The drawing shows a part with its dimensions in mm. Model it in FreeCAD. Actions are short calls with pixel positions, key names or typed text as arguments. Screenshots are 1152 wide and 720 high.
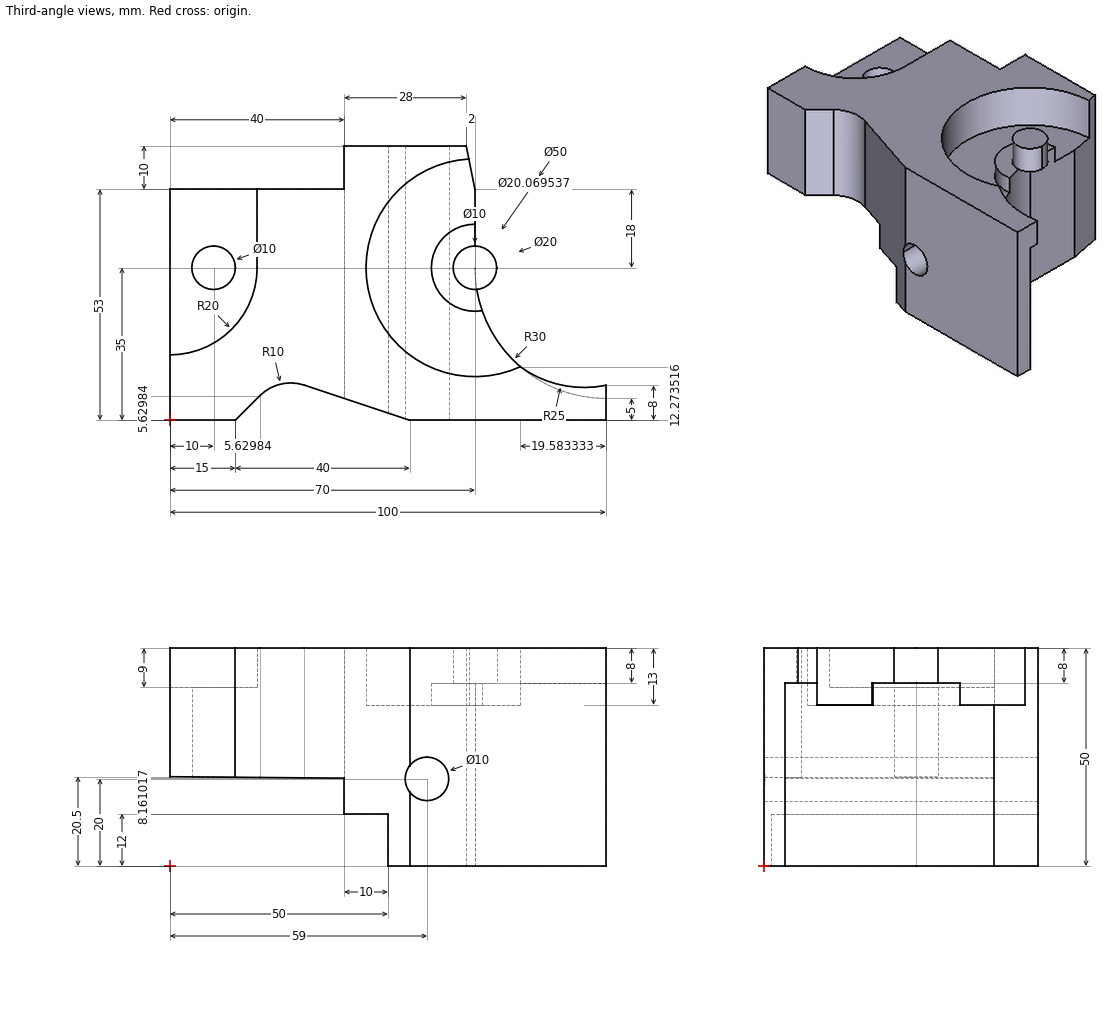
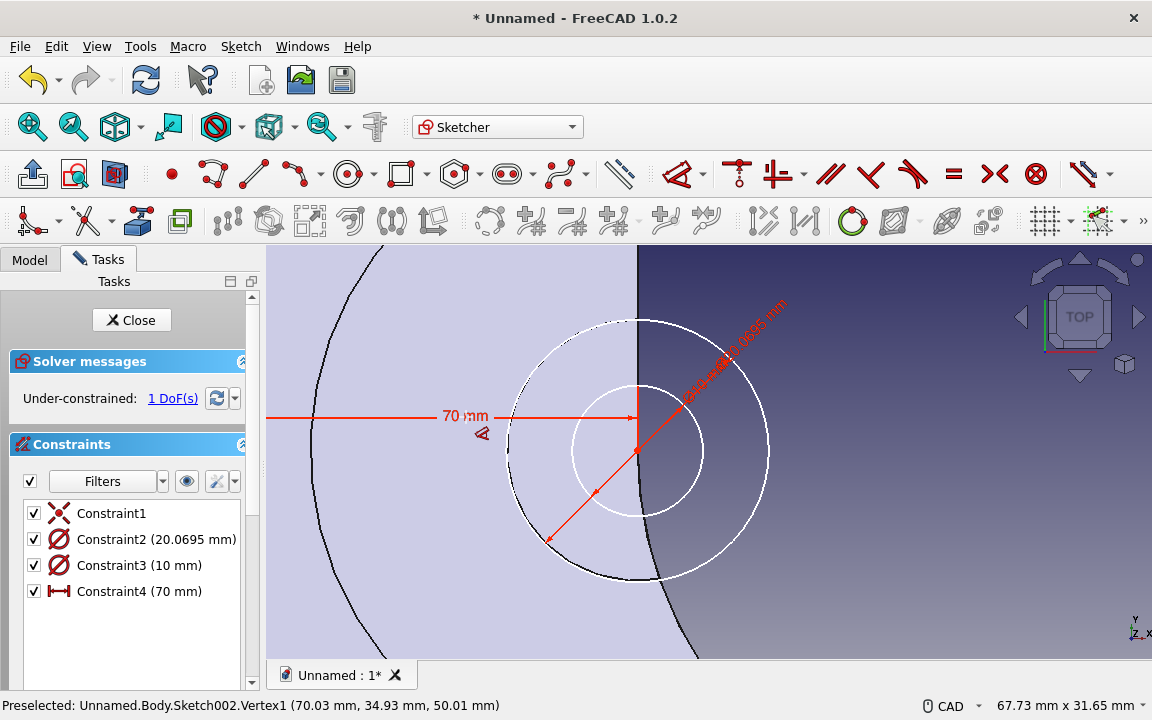
click(638, 451)
click(672, 541)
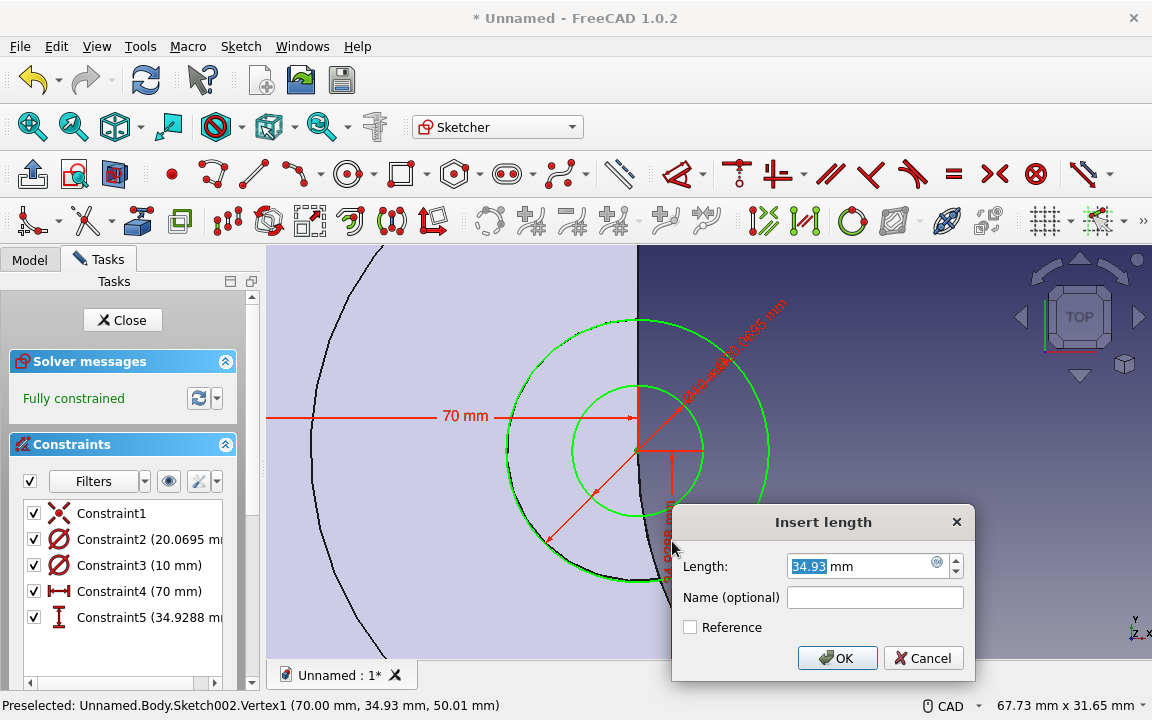
text(35)
key(Return)
key(Escape)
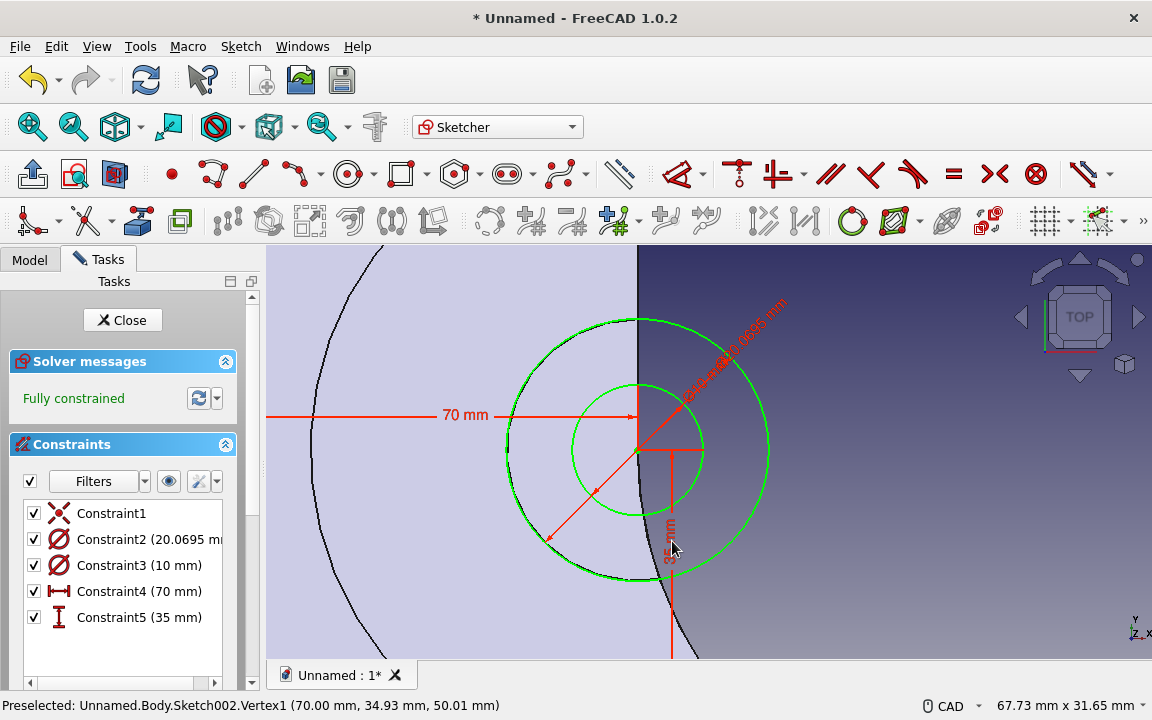
click(123, 320)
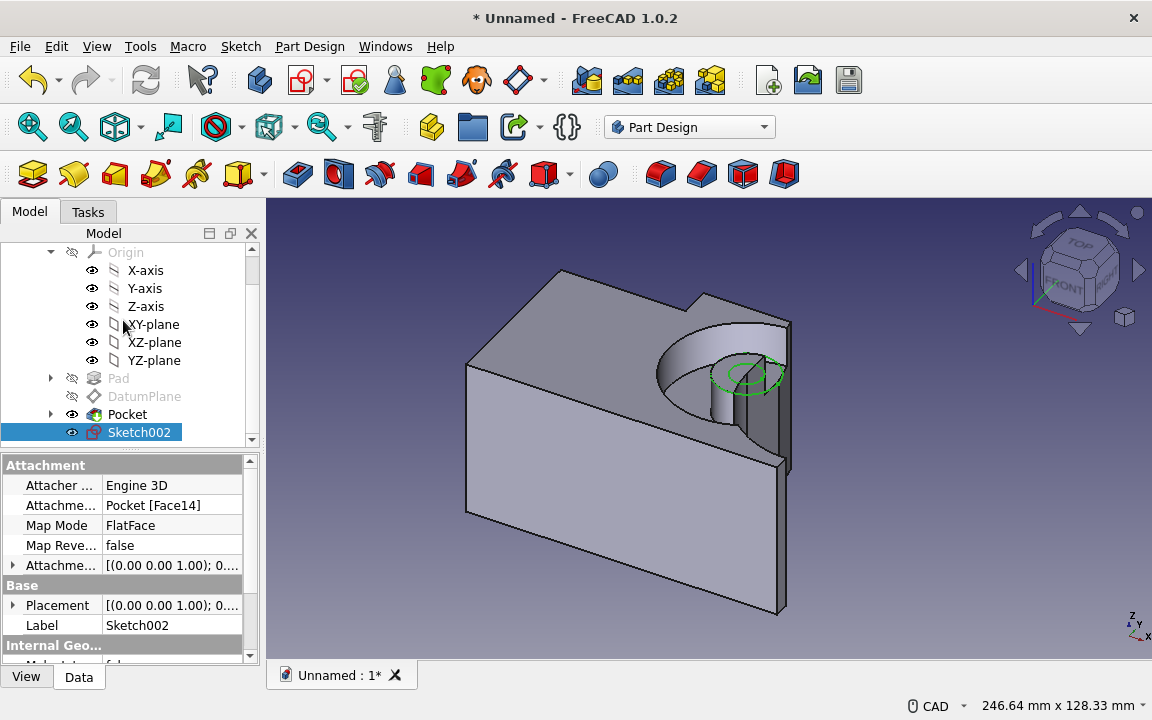
click(298, 174)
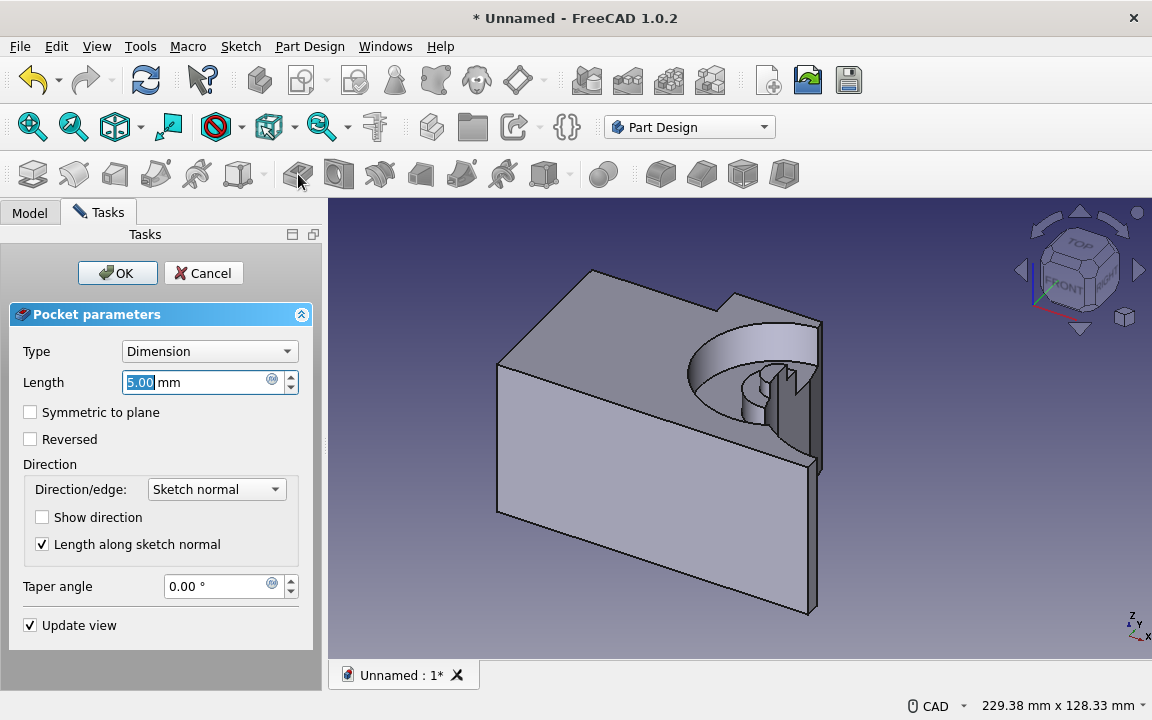
text(8)
key(Tab)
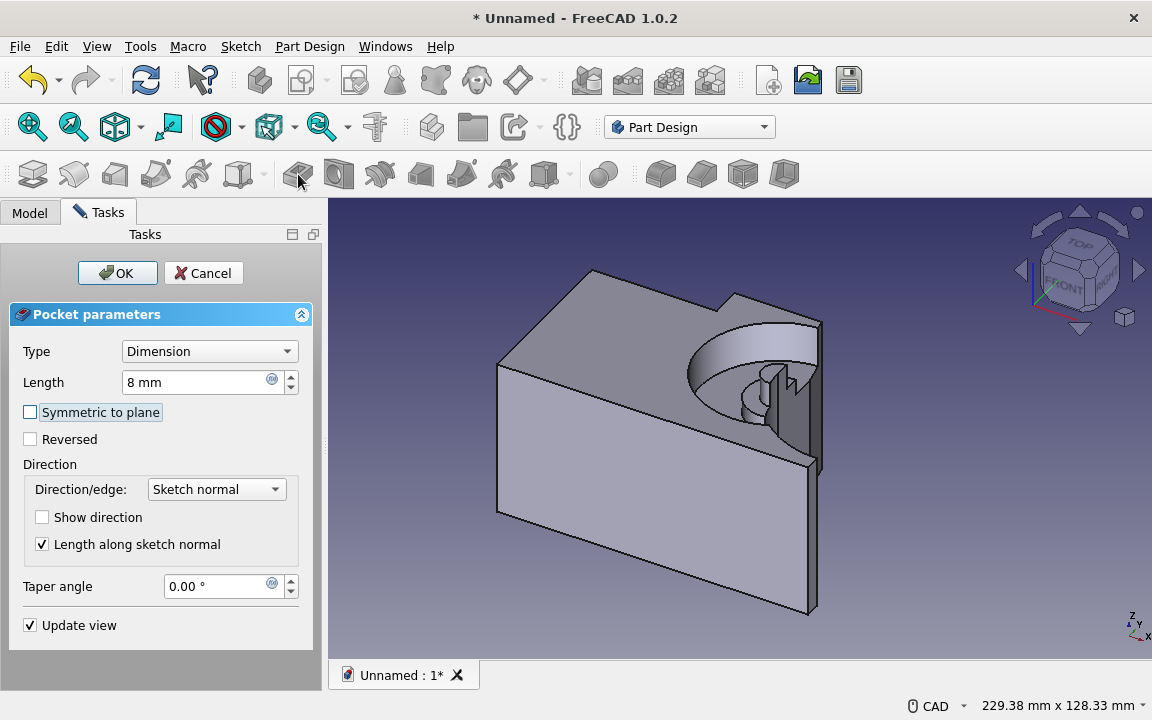
click(118, 273)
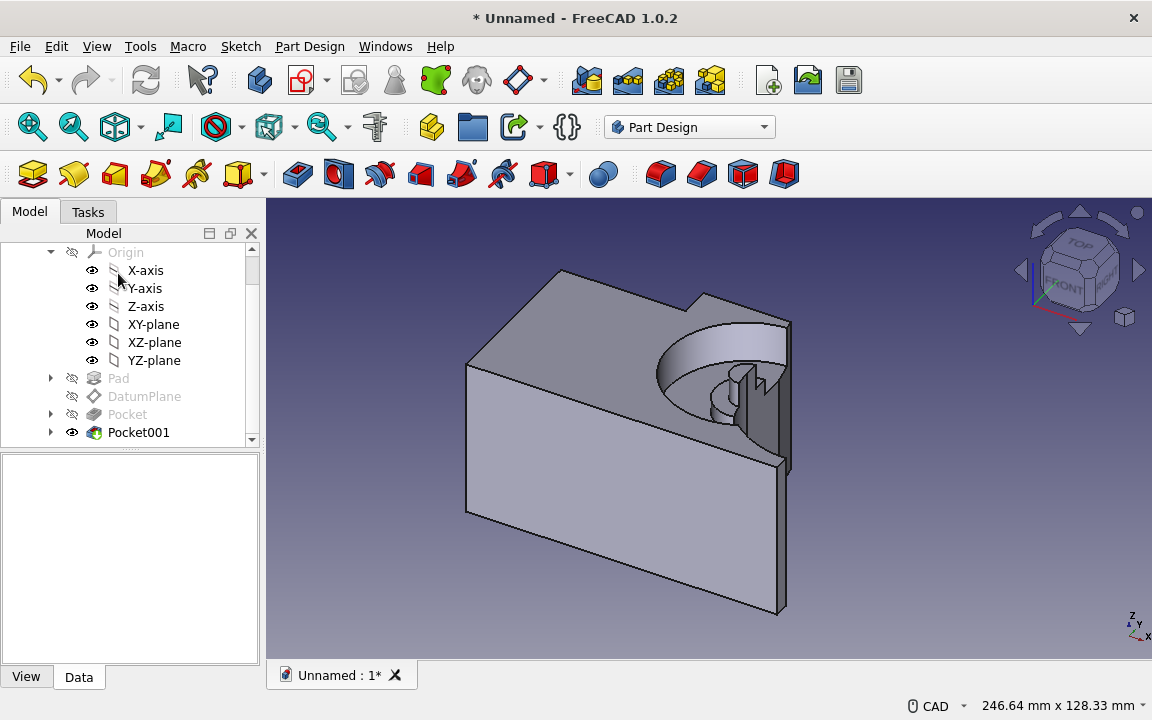
click(589, 329)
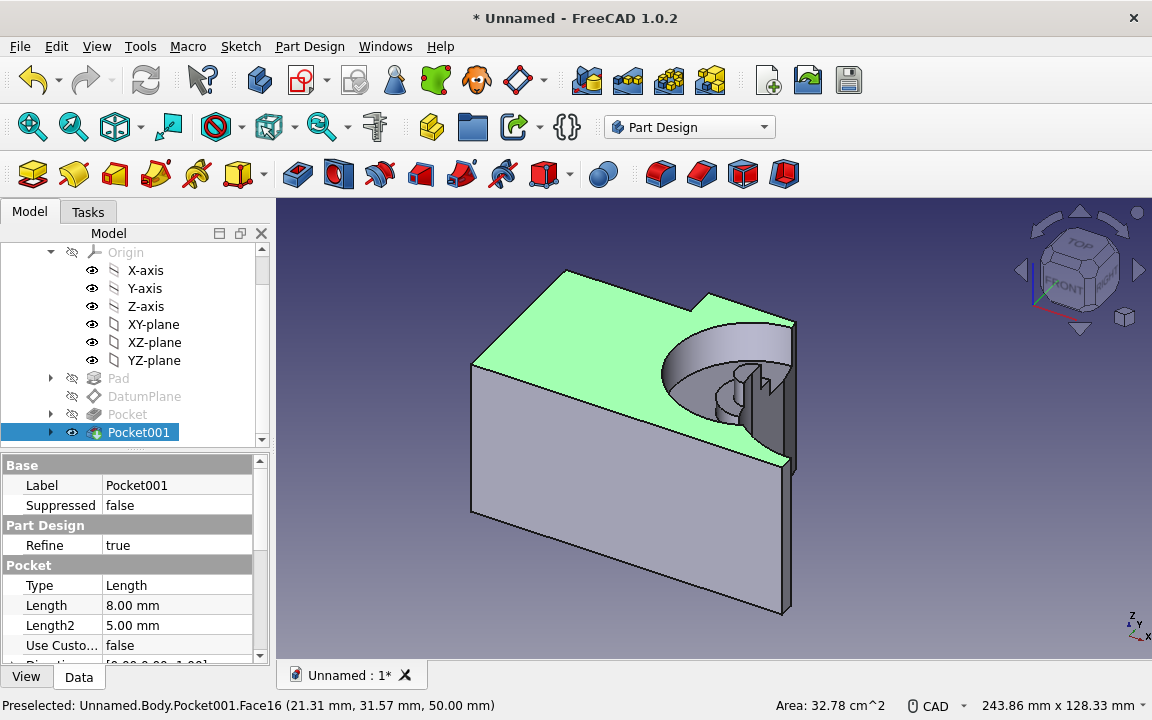
click(300, 80)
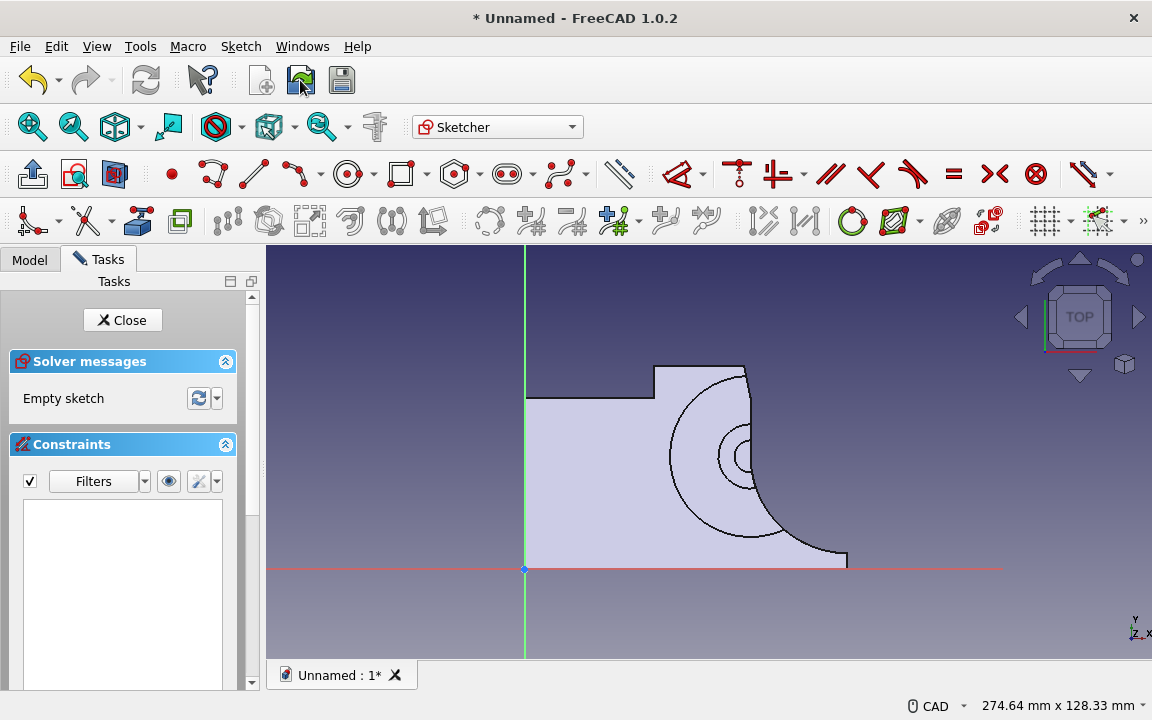
scroll(768, 457, up, 10)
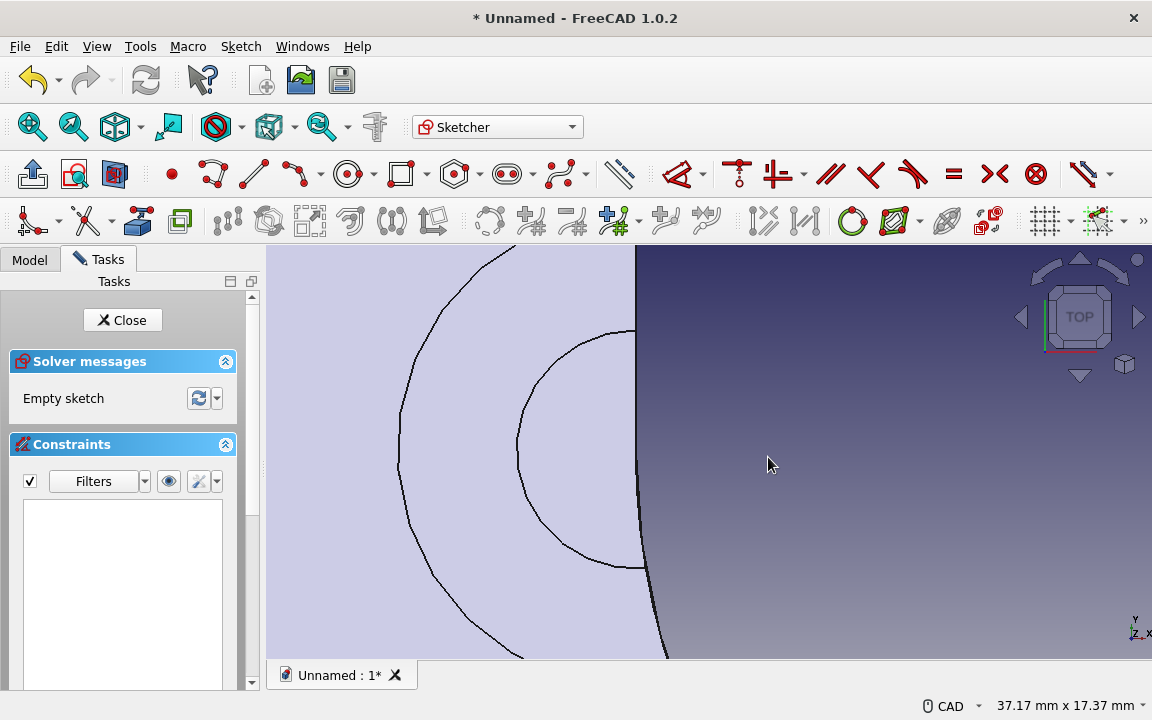
key(g)
key(c)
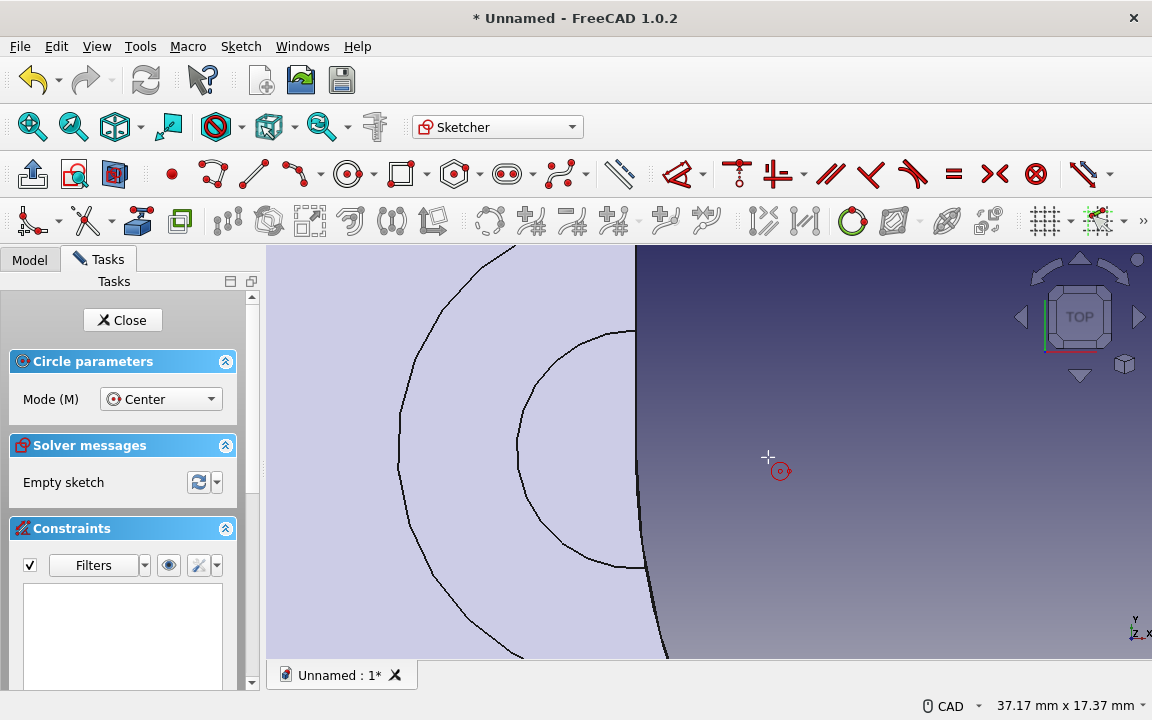
click(636, 450)
click(720, 365)
key(Escape)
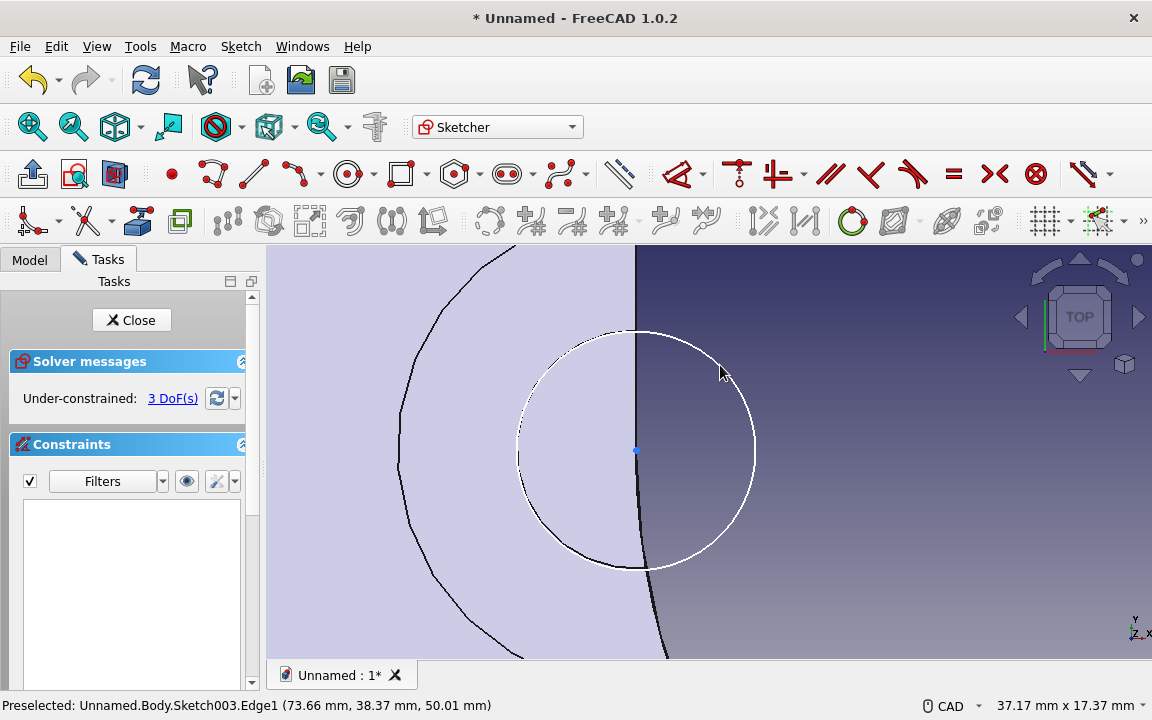
key(d)